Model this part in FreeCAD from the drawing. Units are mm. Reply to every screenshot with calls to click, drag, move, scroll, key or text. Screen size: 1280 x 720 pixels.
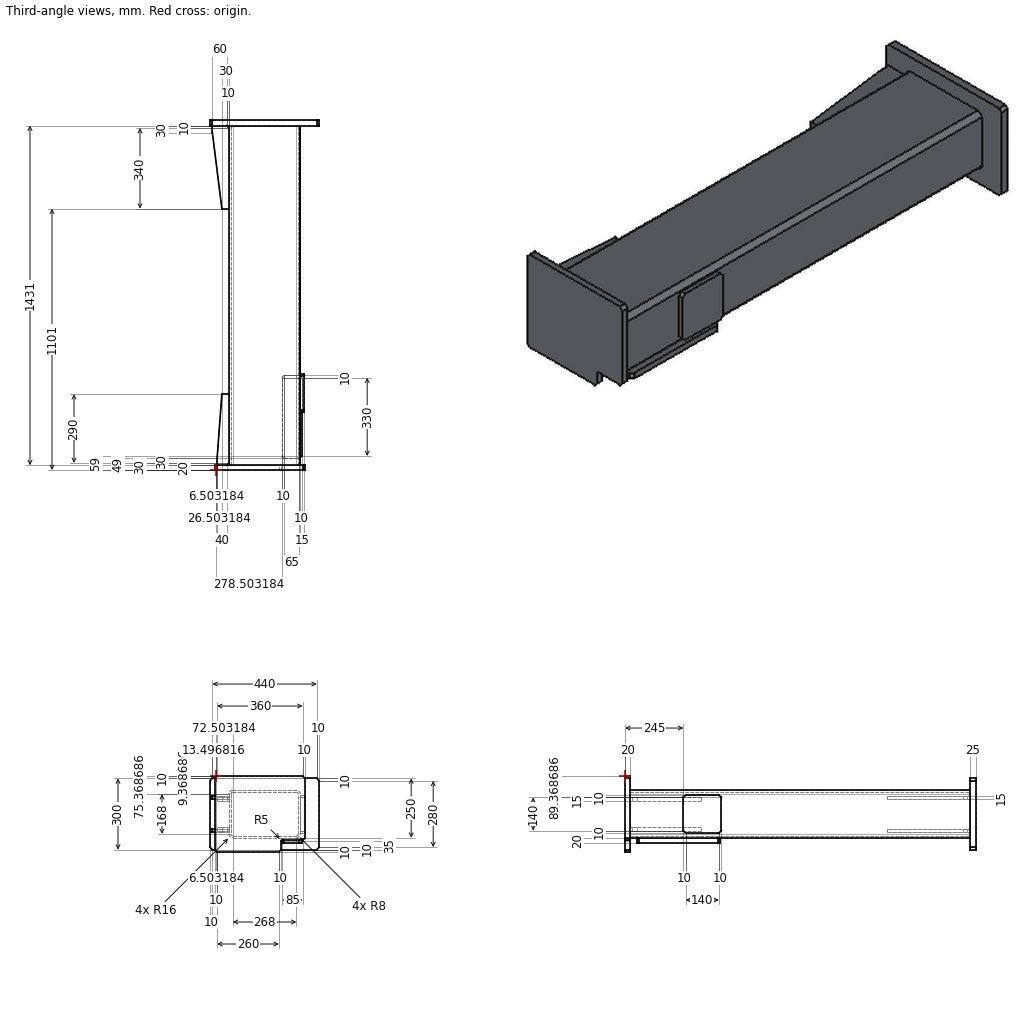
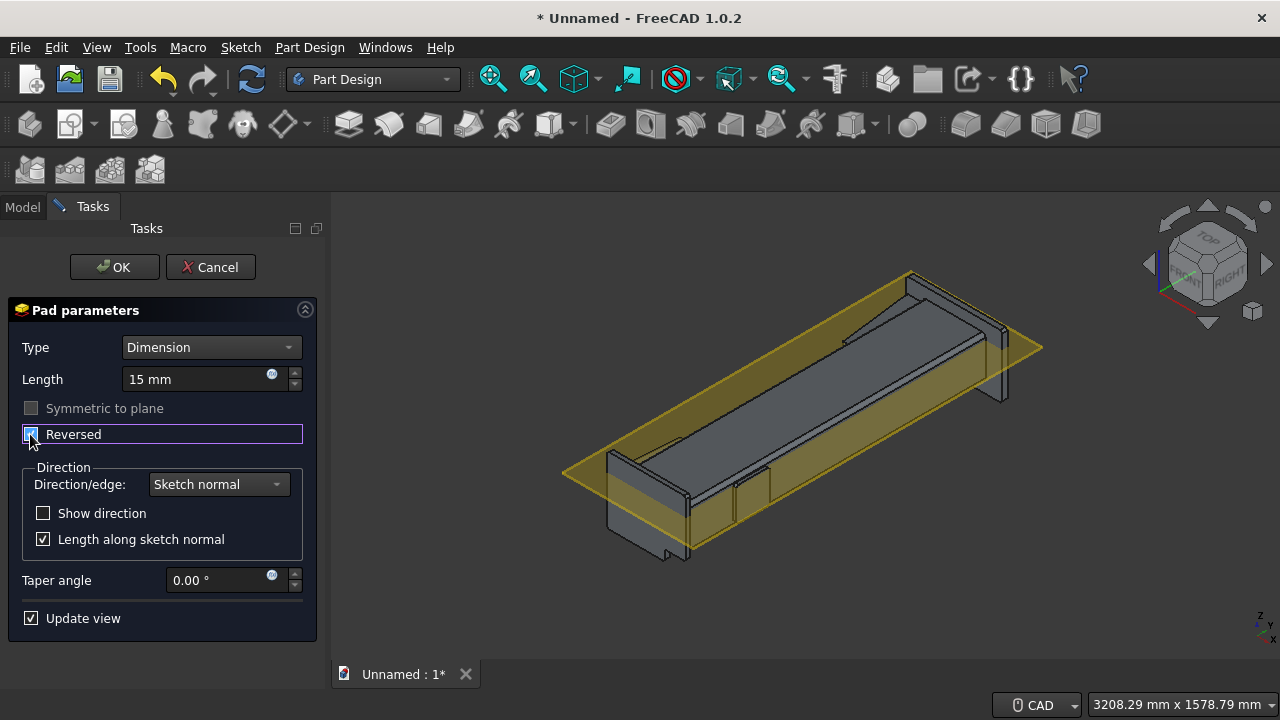
click(115, 267)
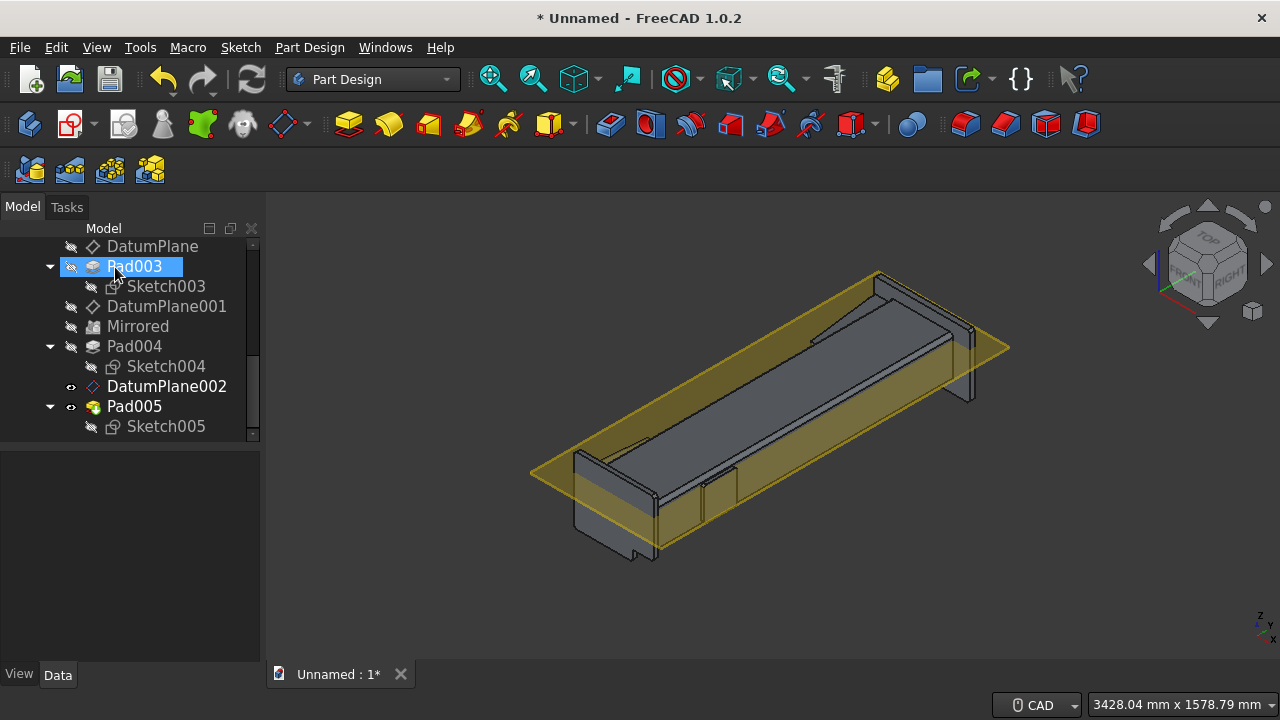
click(116, 387)
key(space)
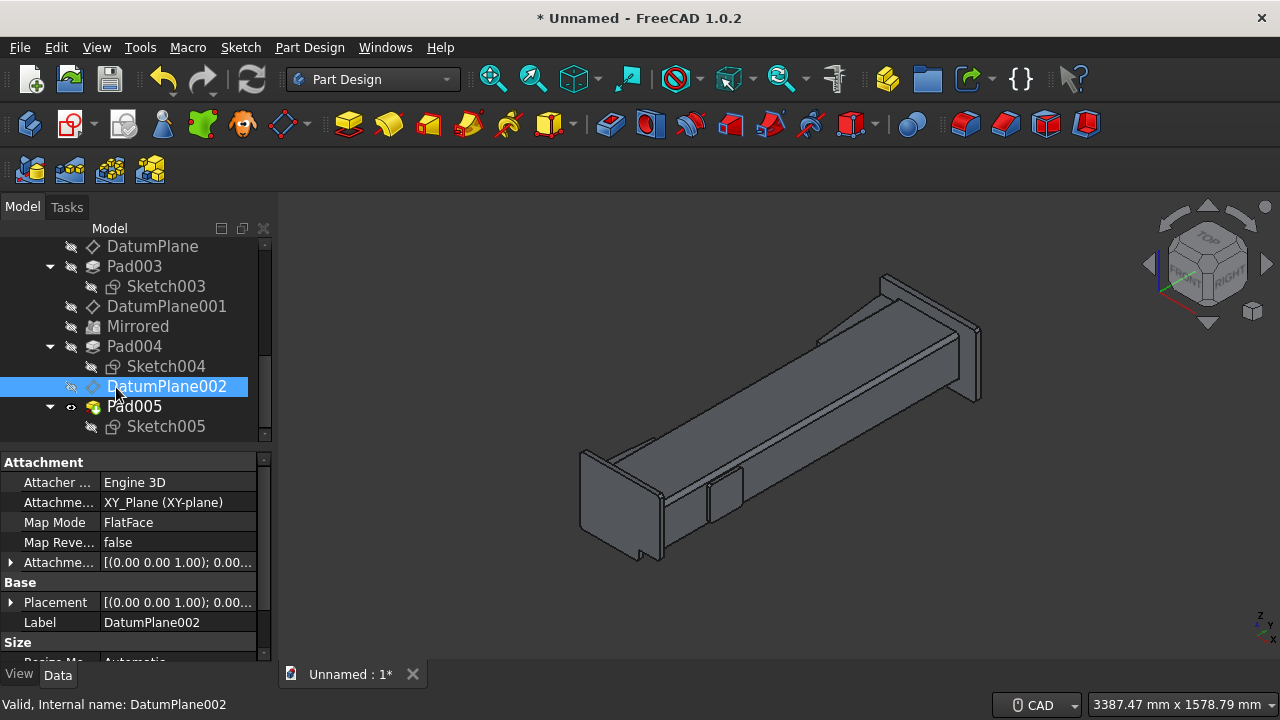
scroll(140, 342, down, 3)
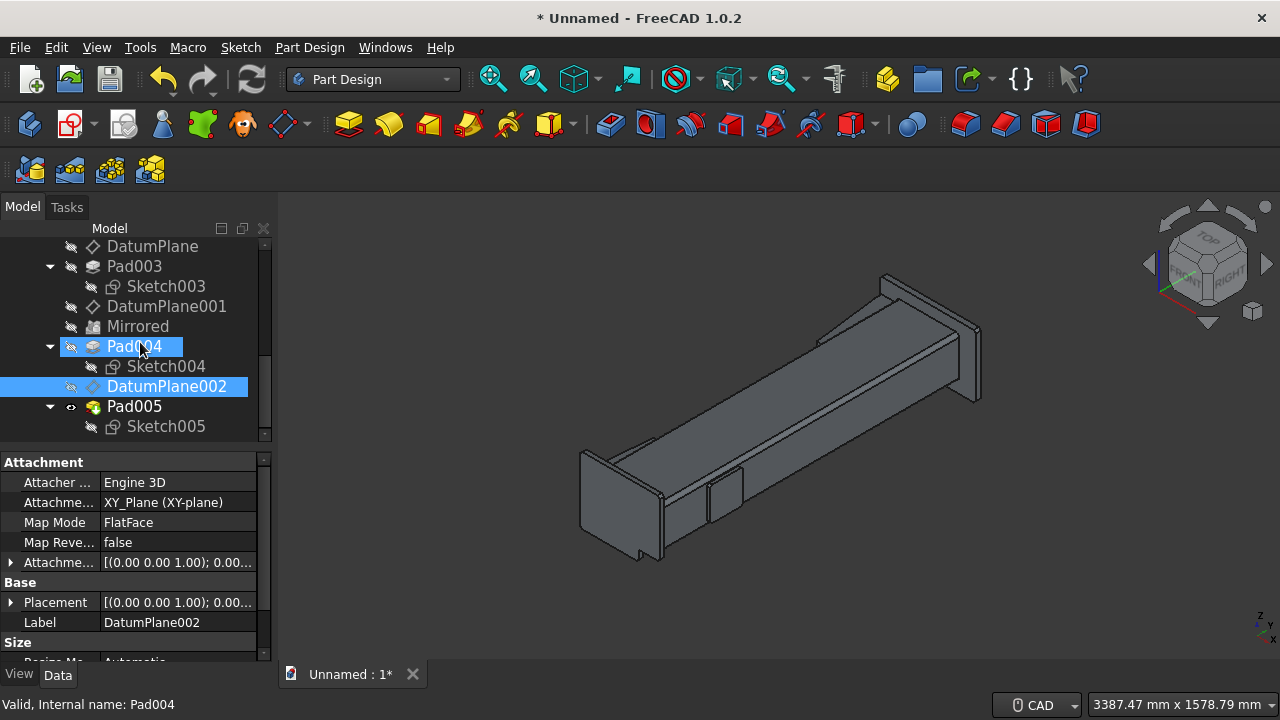
scroll(140, 342, up, 15)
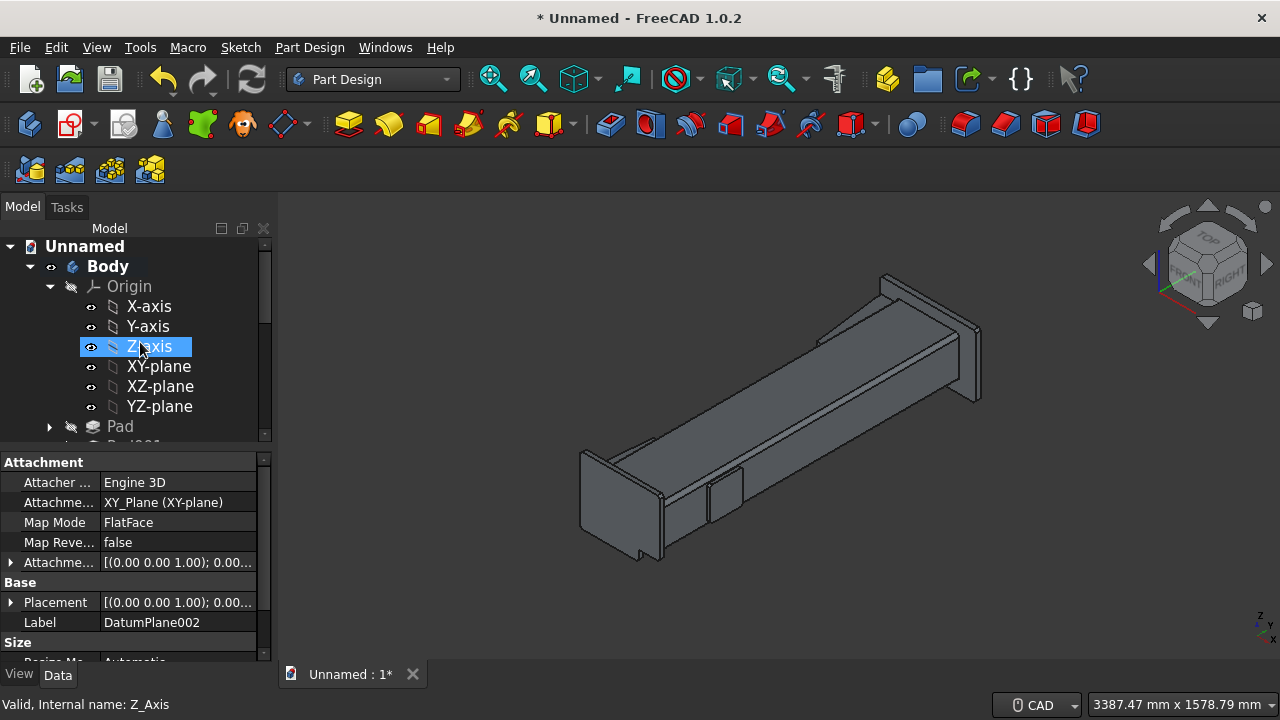
click(136, 367)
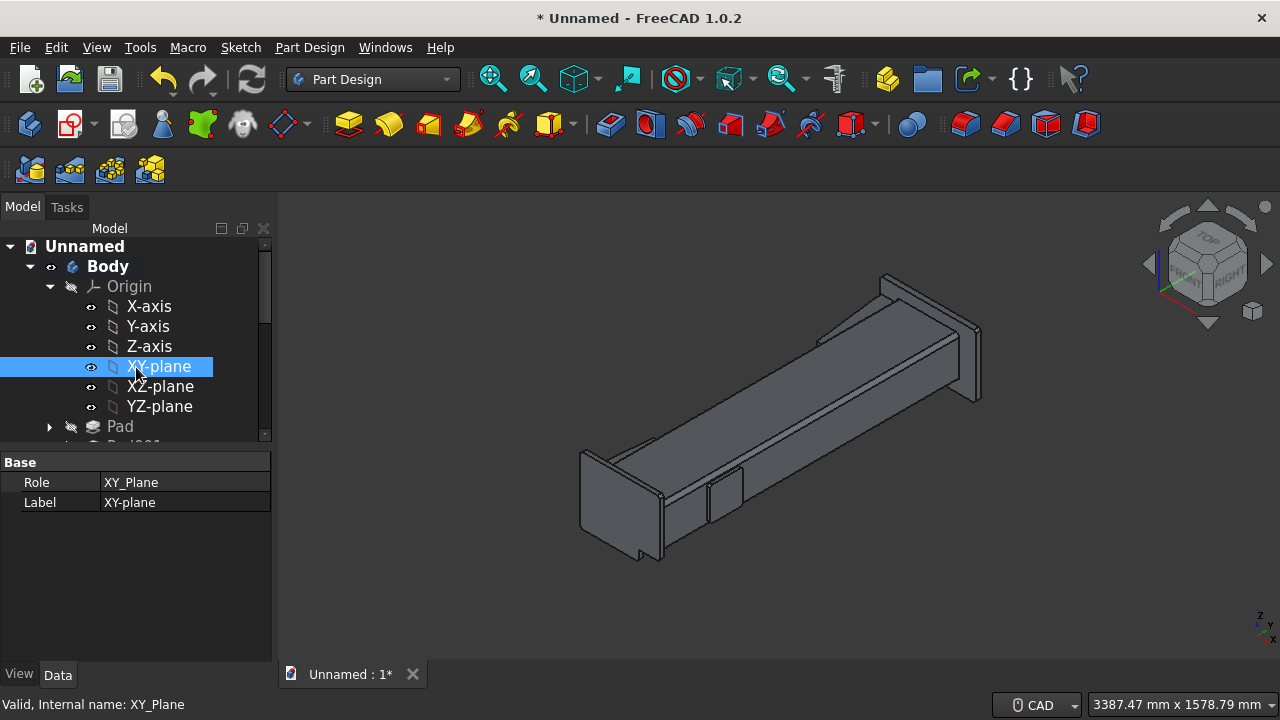
click(284, 124)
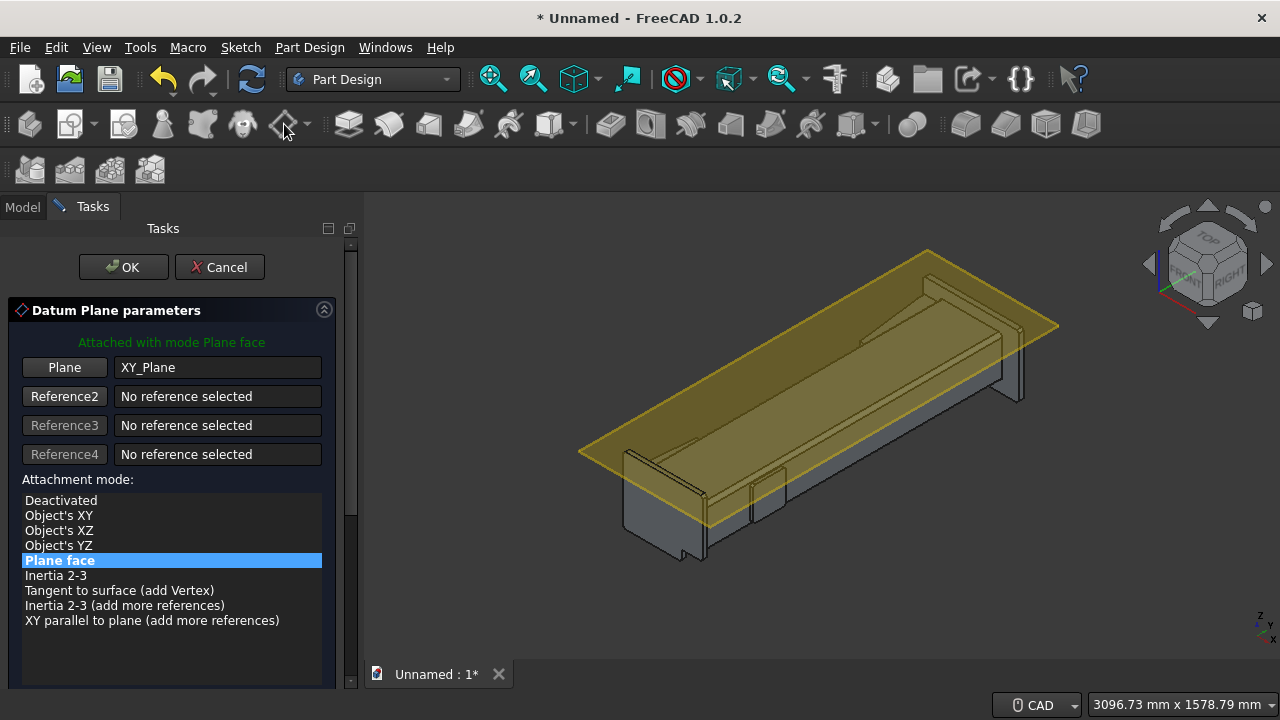
scroll(351, 463, down, 3)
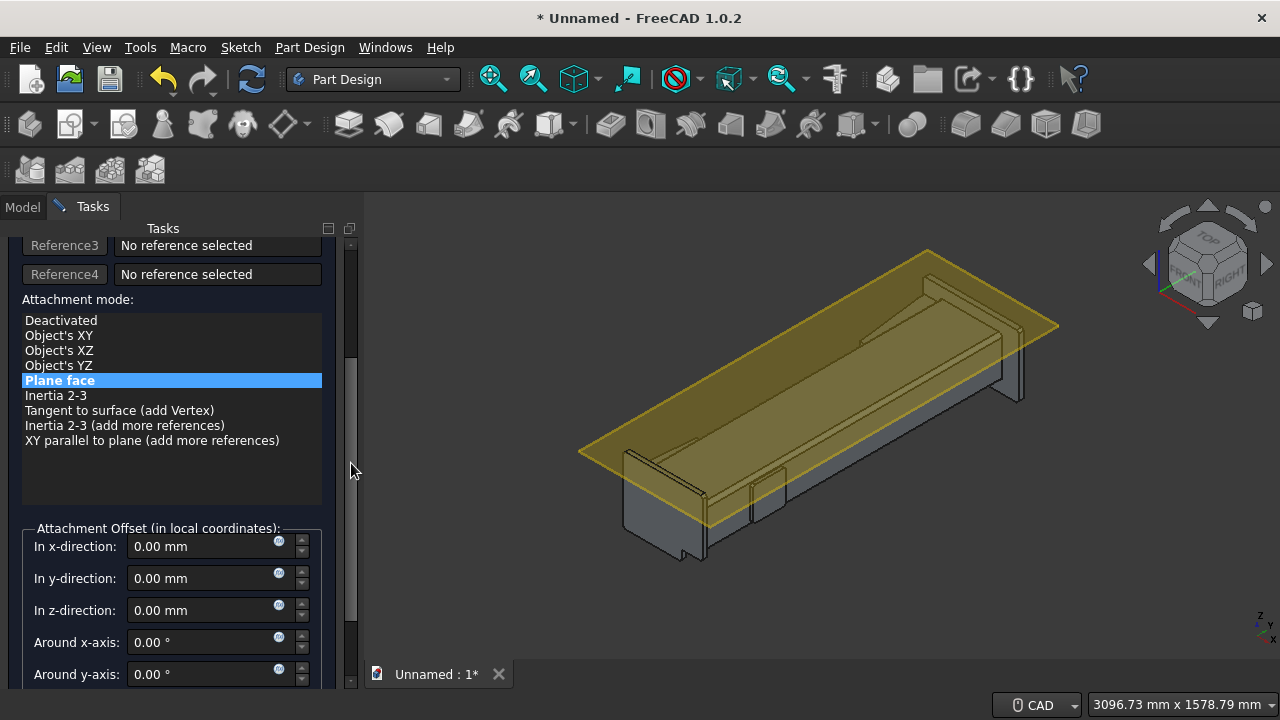
triple_click(210, 610)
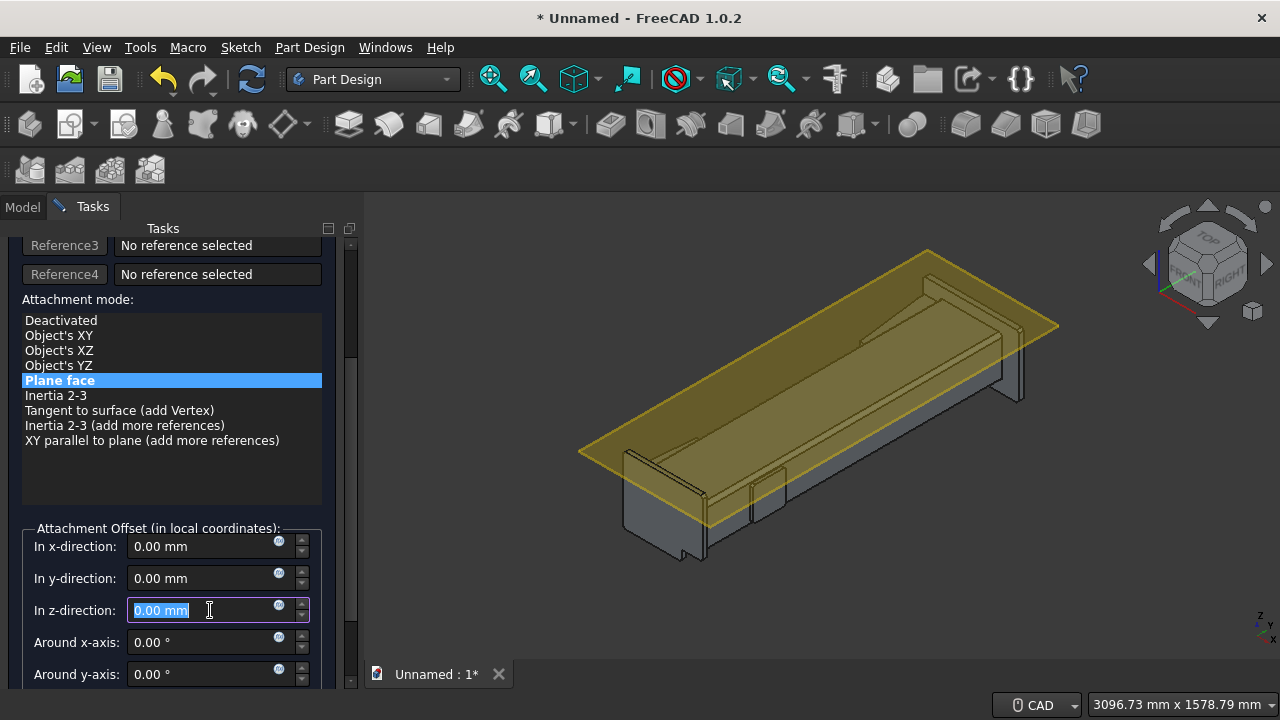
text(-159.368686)
key(Tab)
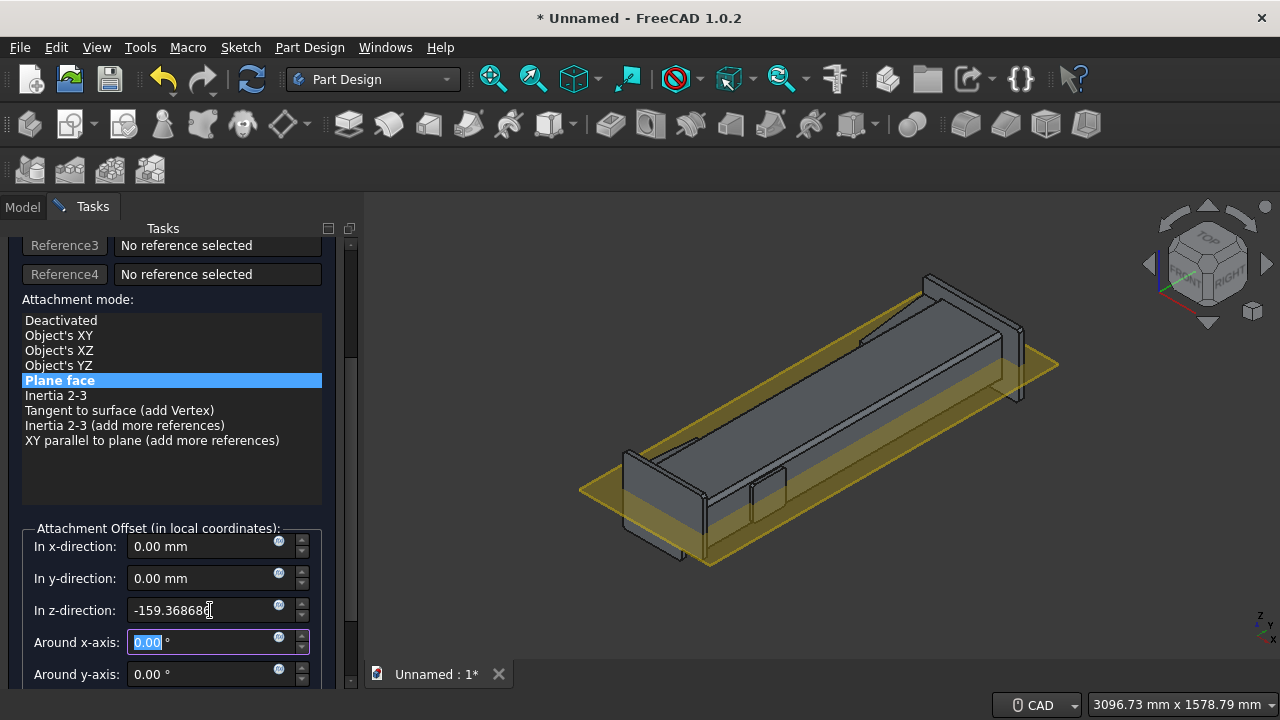
scroll(351, 463, up, 4)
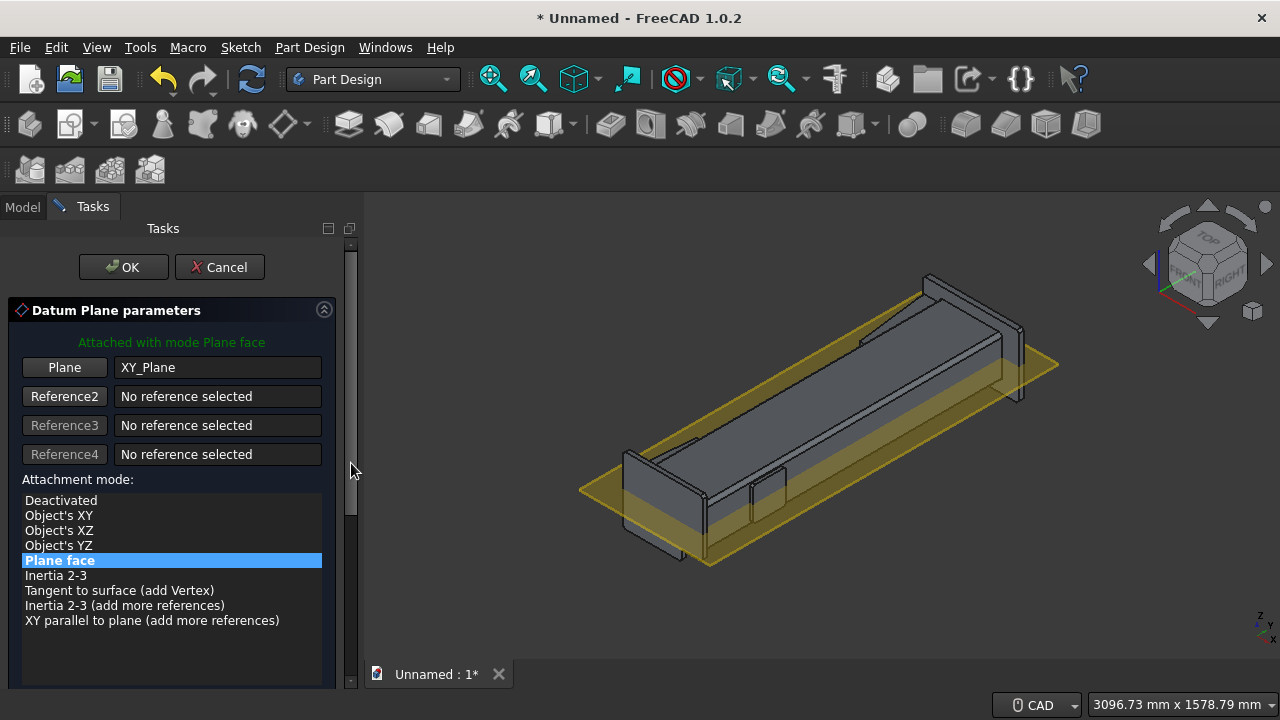
click(124, 267)